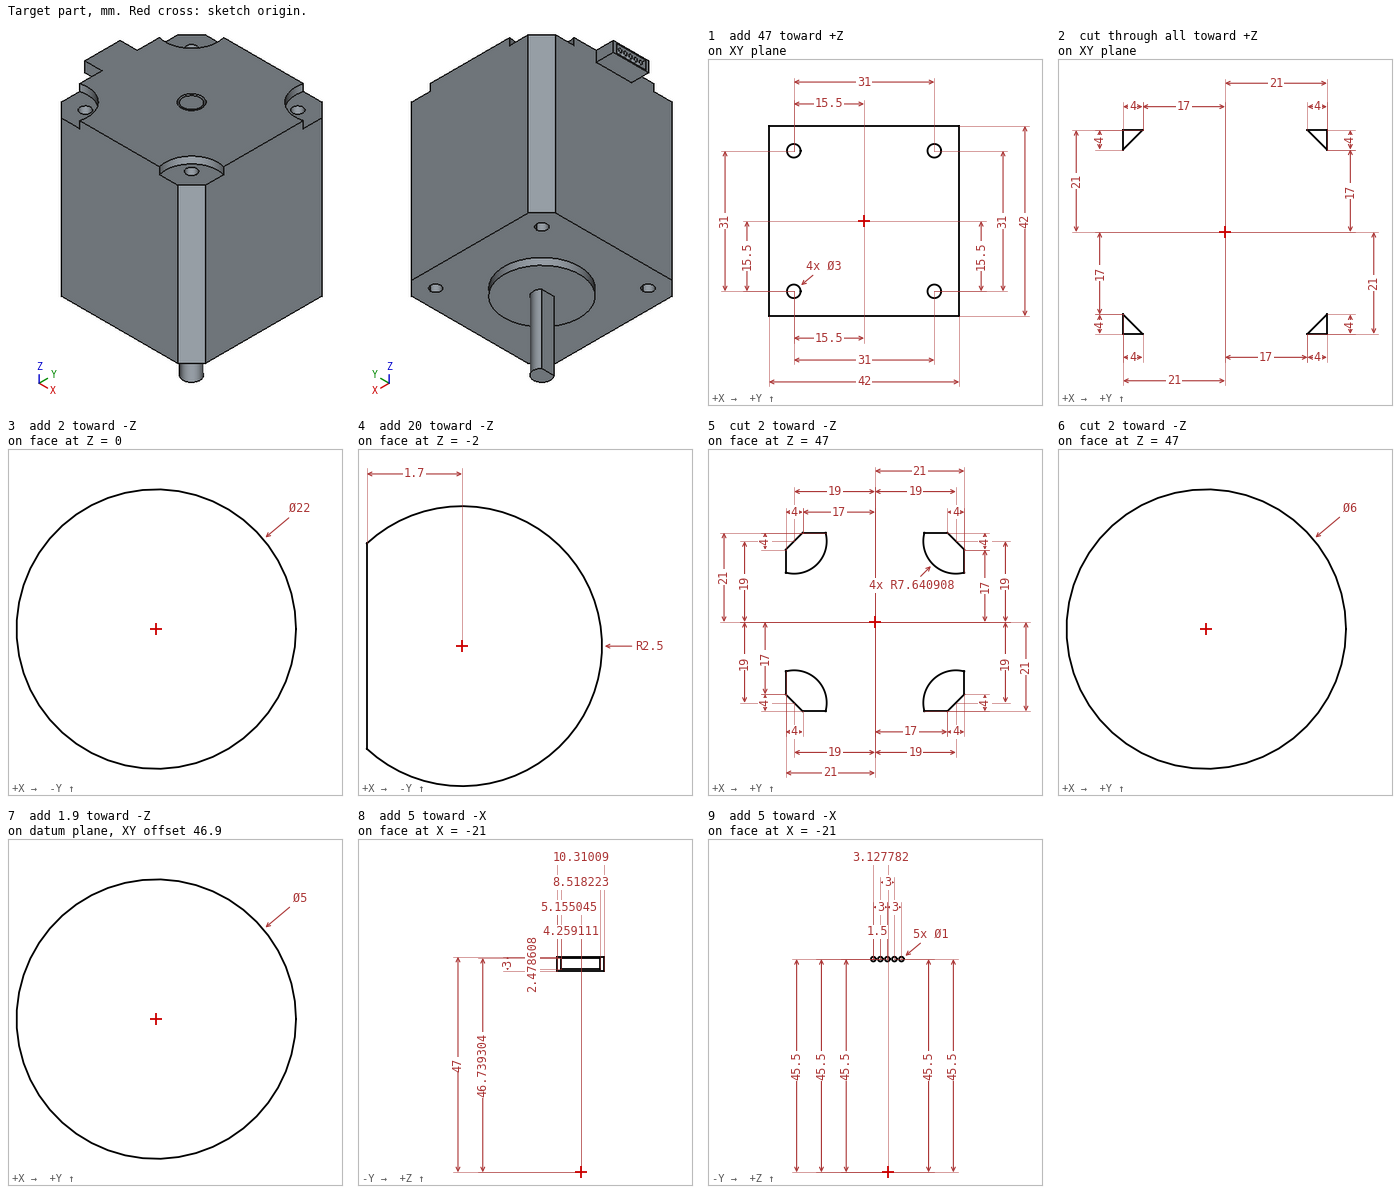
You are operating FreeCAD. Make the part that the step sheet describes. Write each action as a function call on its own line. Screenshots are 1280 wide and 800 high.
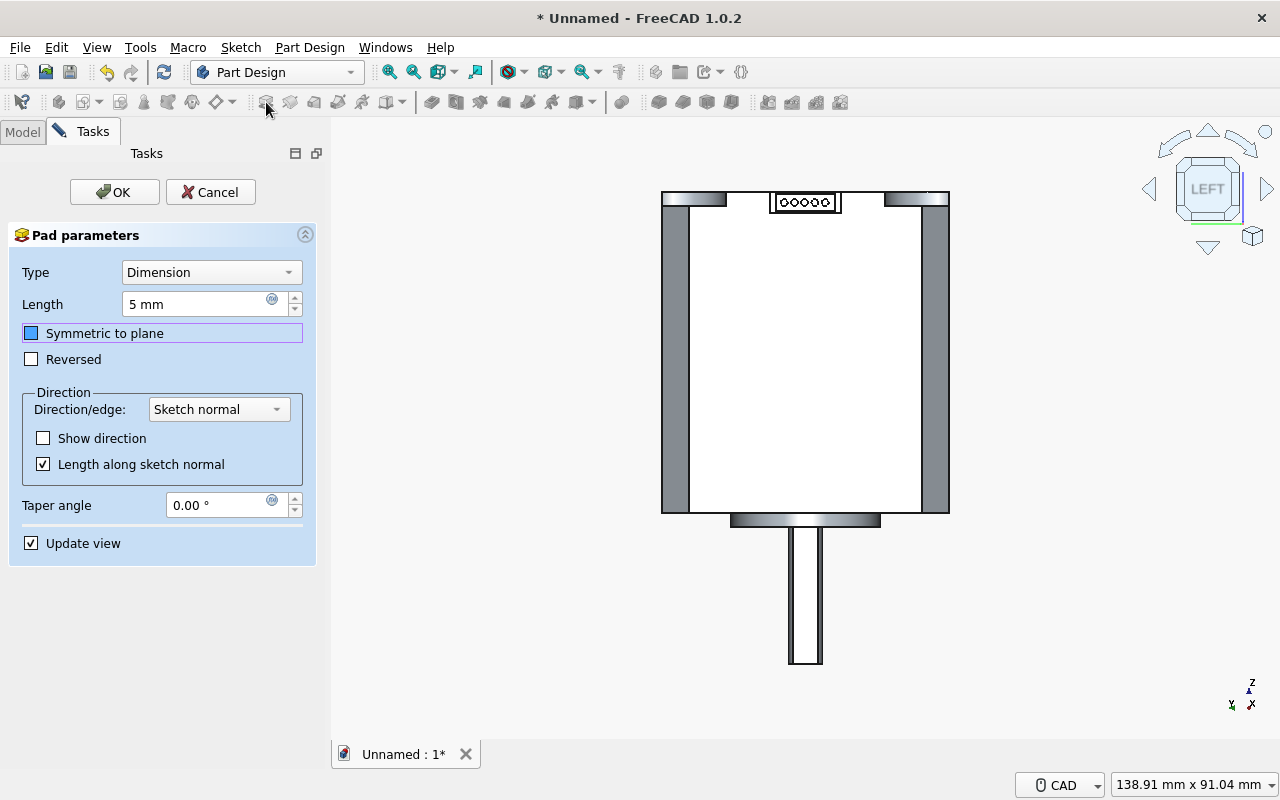
click(115, 192)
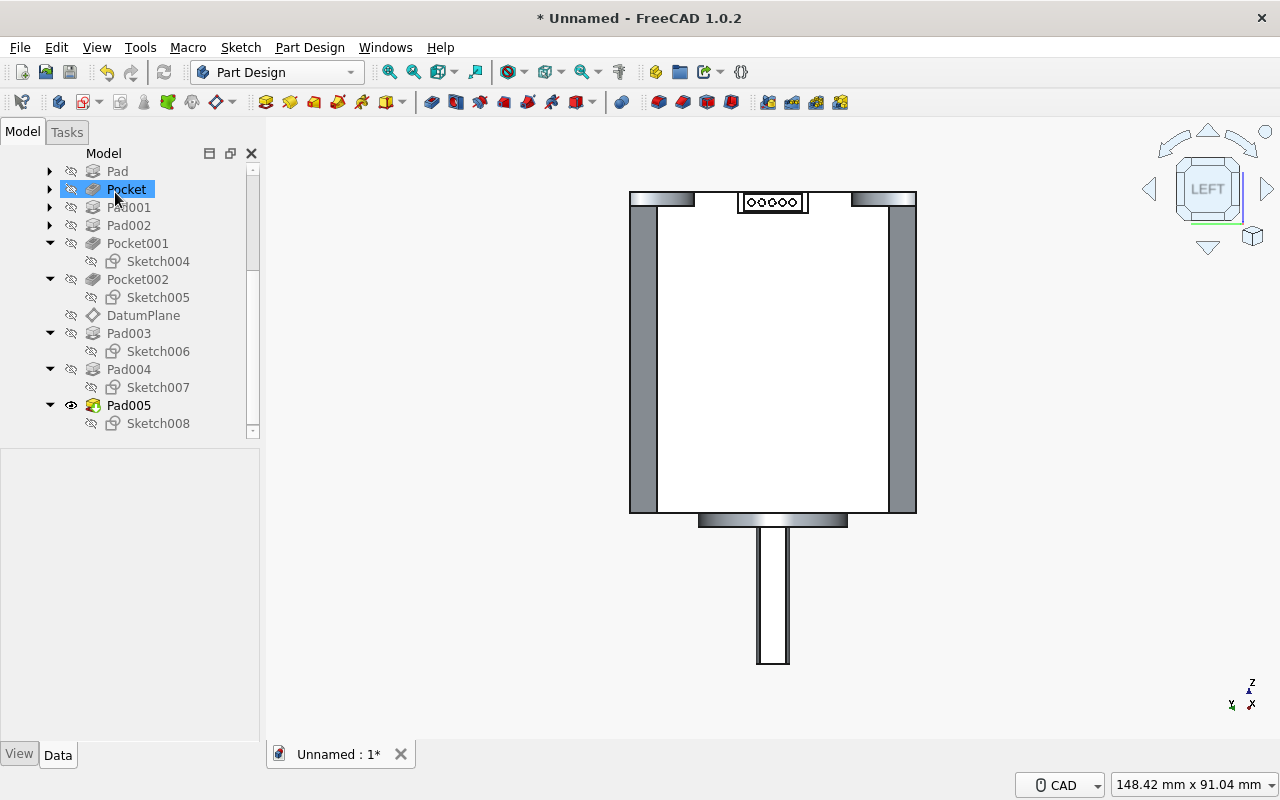
key(0)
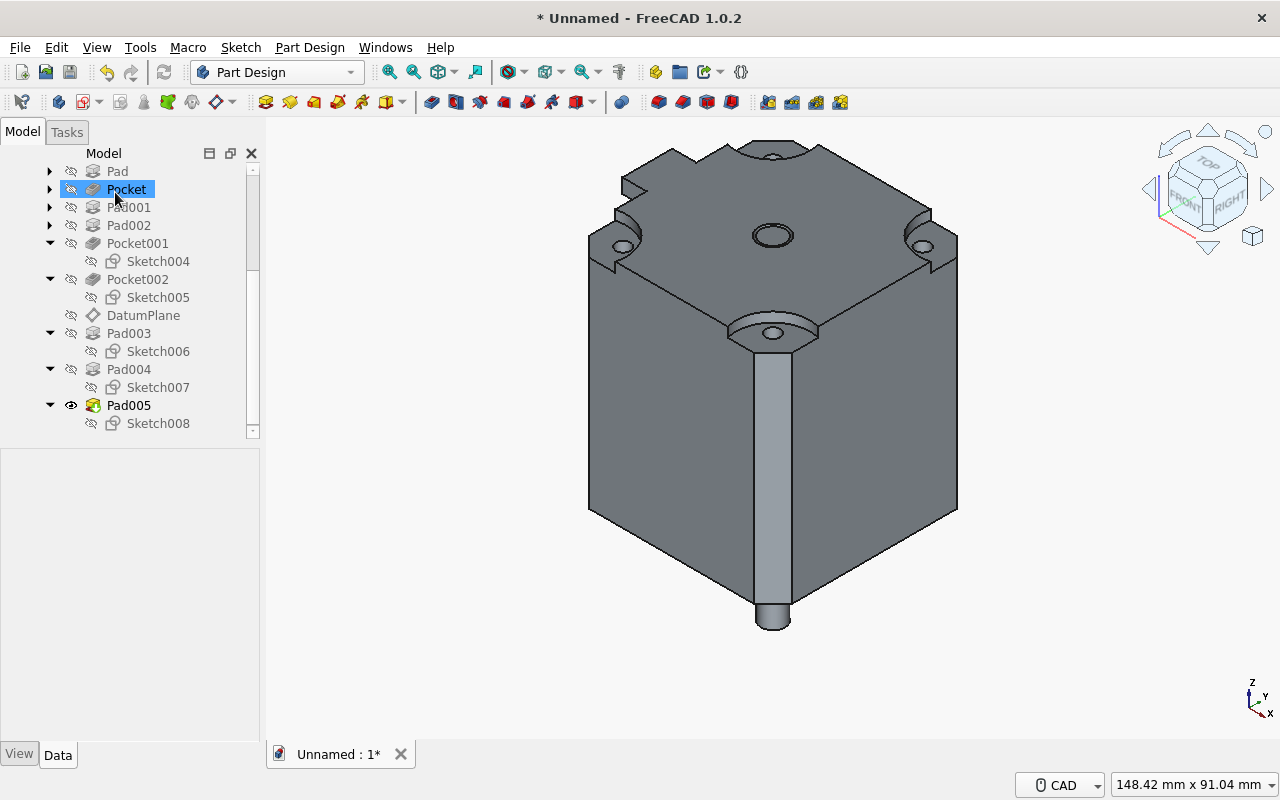
click(390, 72)